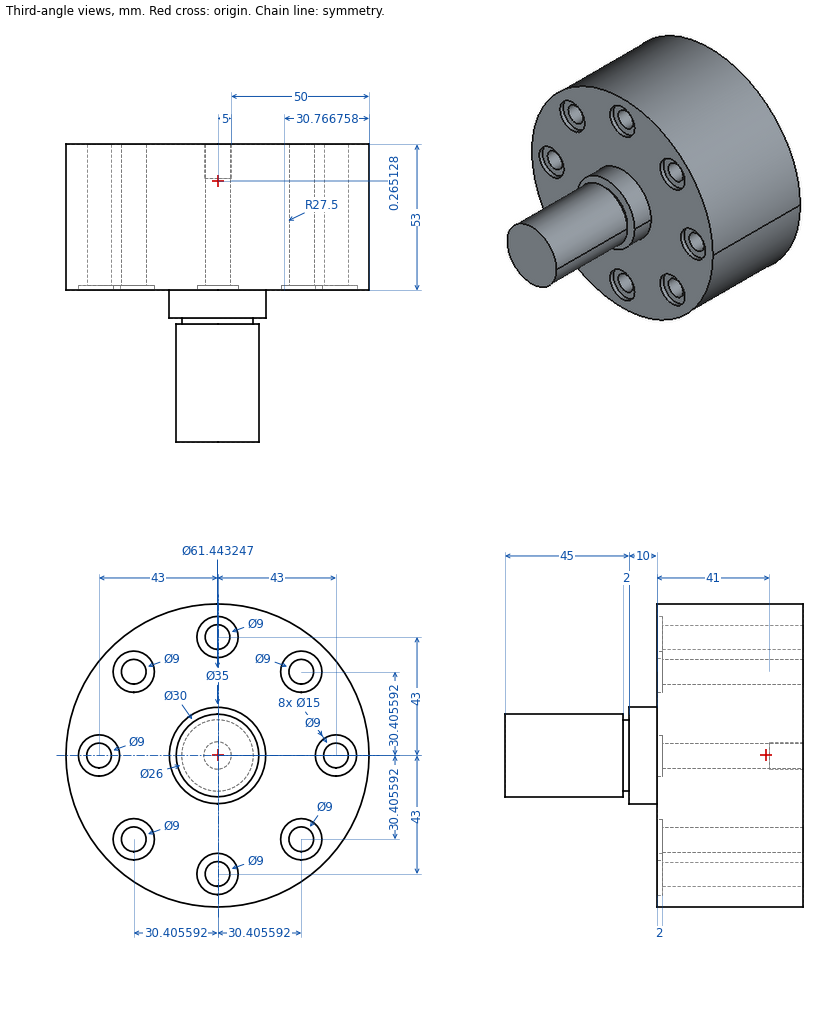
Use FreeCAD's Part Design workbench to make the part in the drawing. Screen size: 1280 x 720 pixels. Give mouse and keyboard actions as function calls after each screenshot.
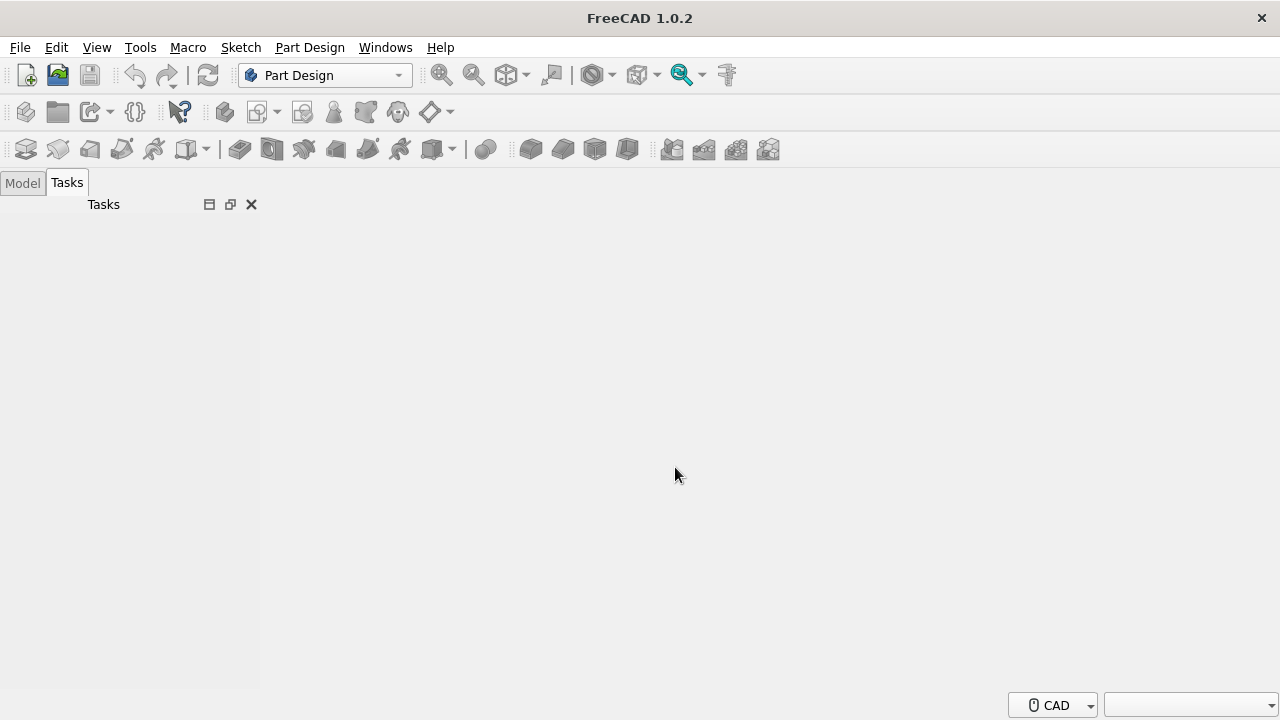
click(26, 76)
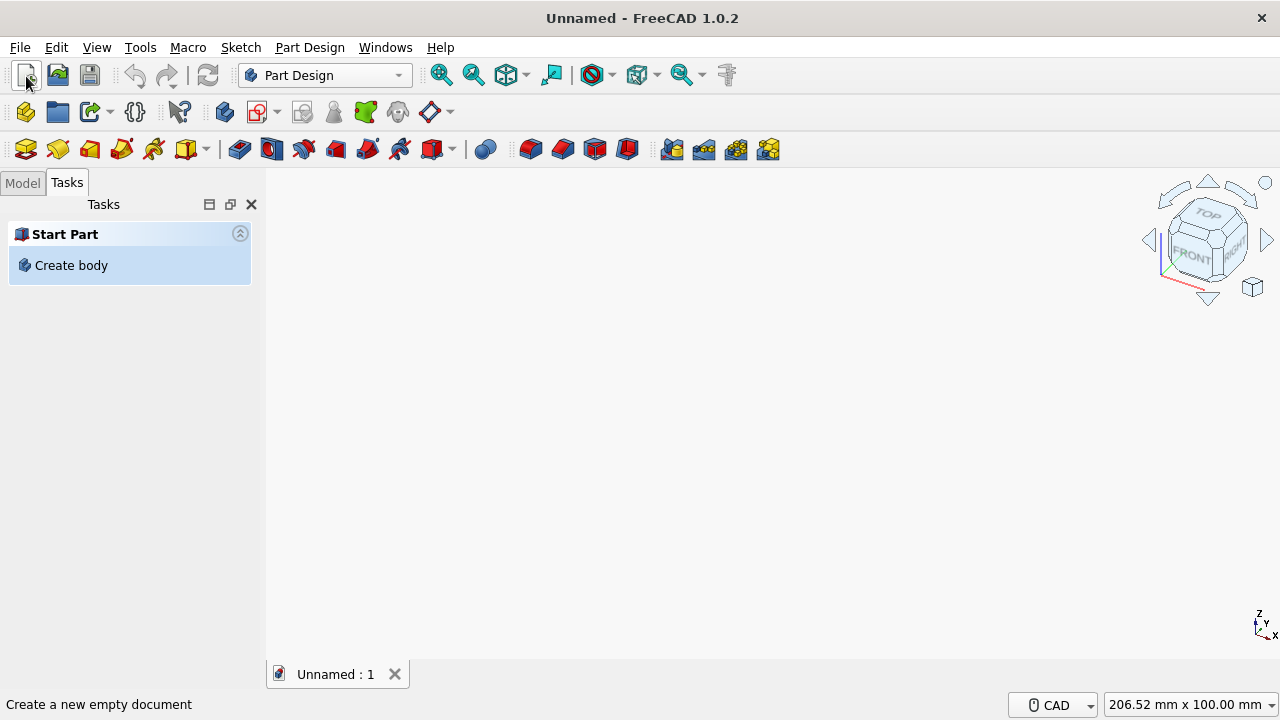
click(258, 112)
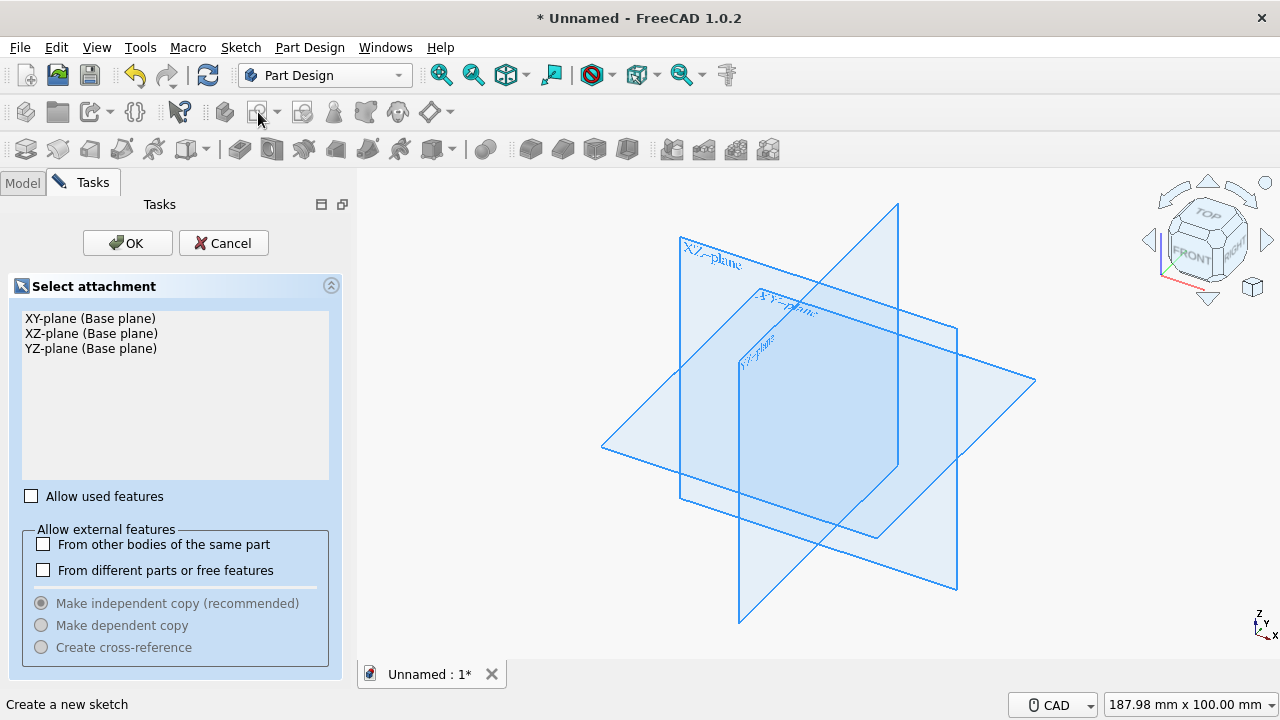
click(82, 318)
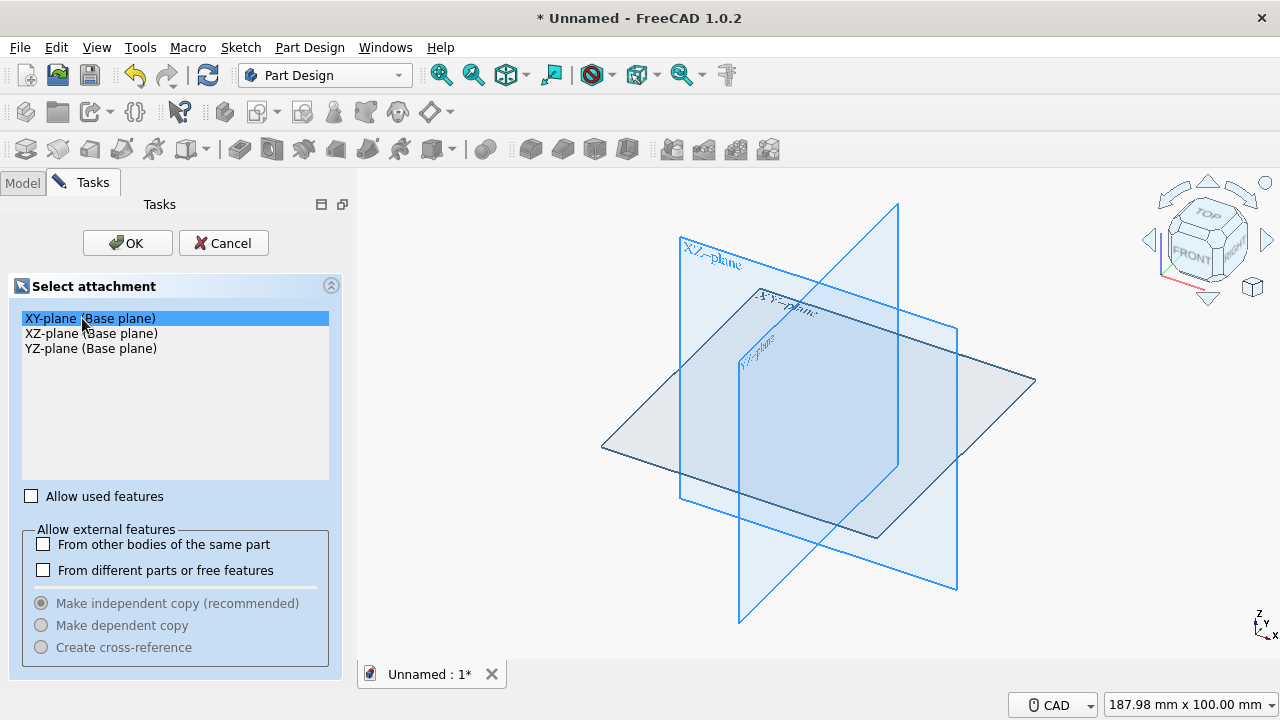
click(128, 243)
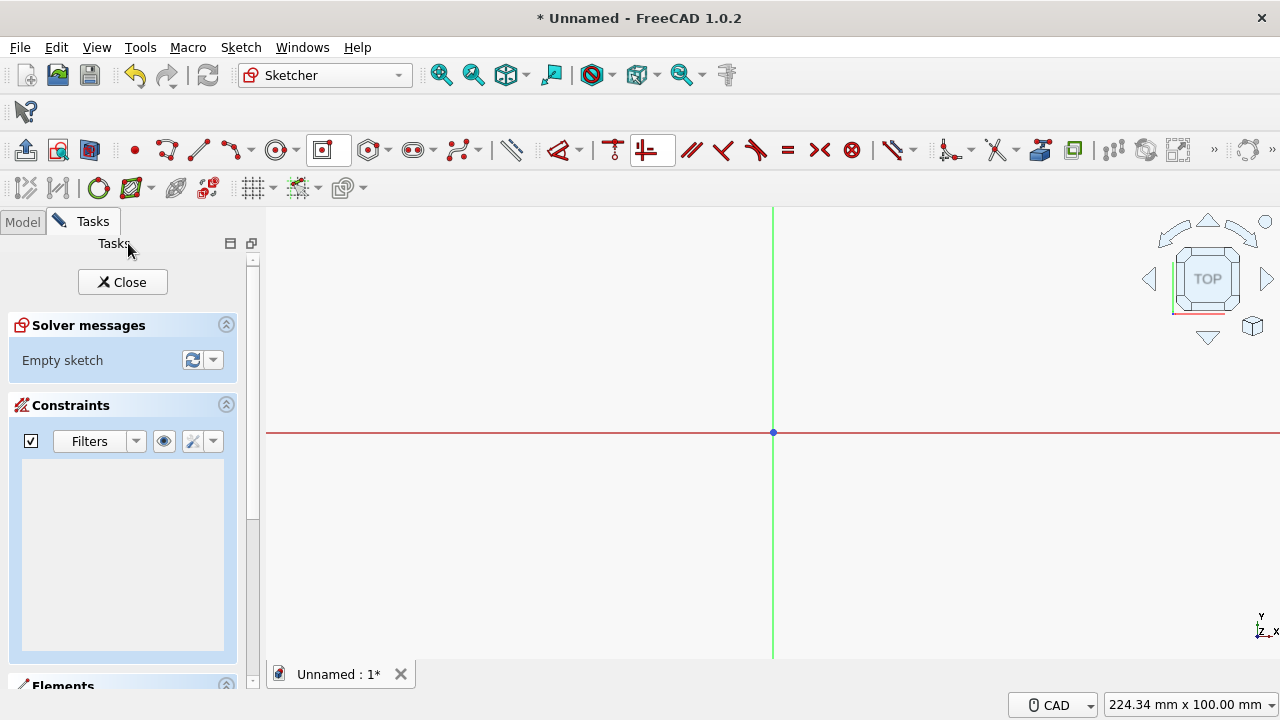
scroll(294, 235, down, 1)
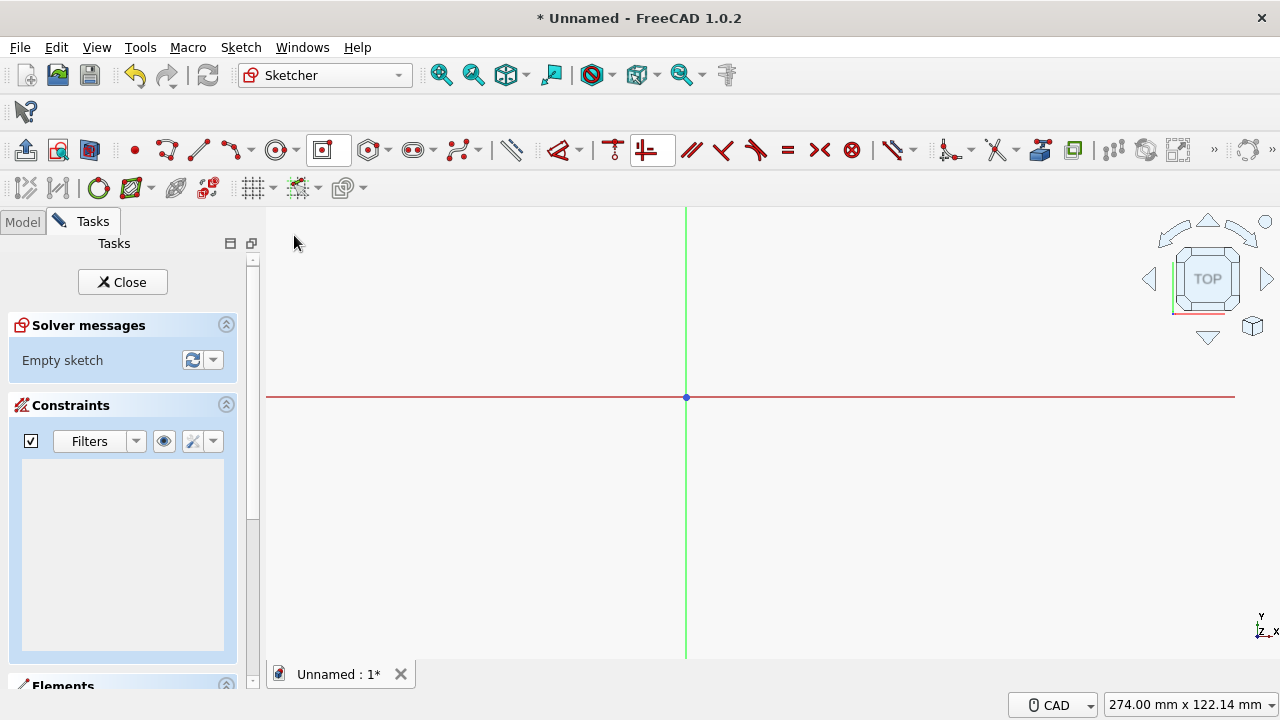
scroll(958, 473, up, 2)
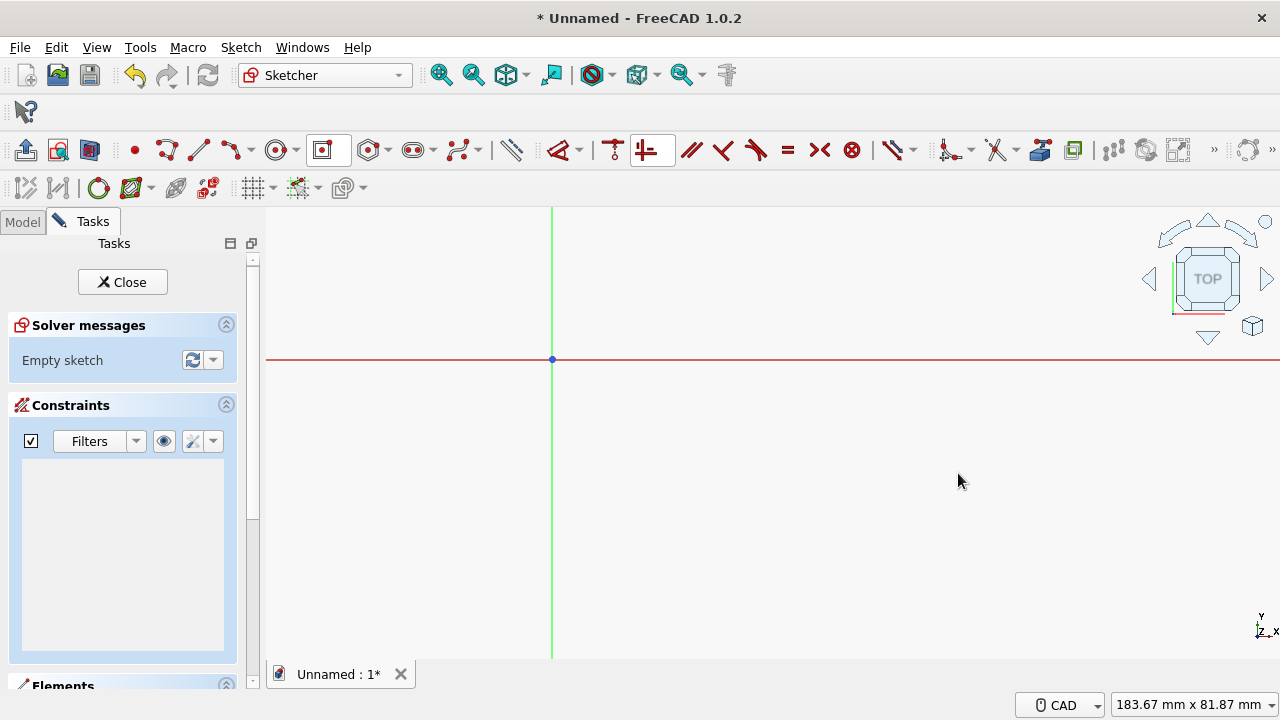
click(168, 150)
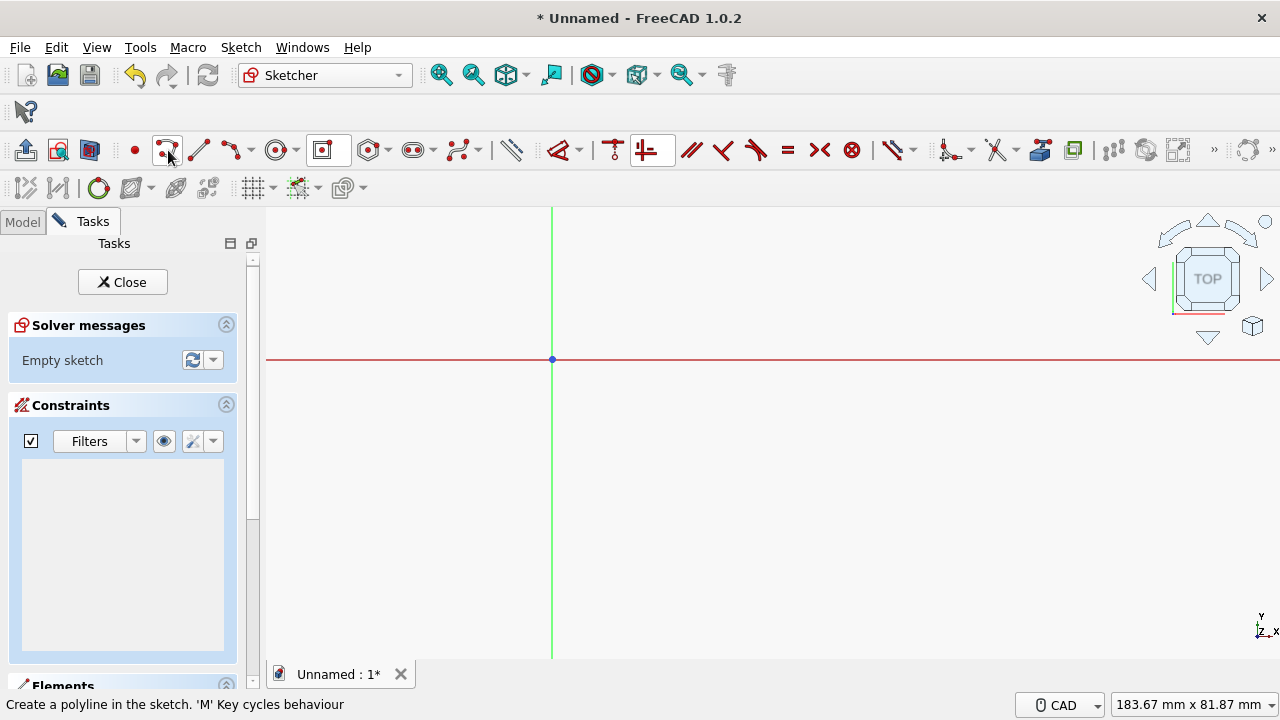
click(686, 579)
click(856, 579)
click(856, 287)
click(580, 287)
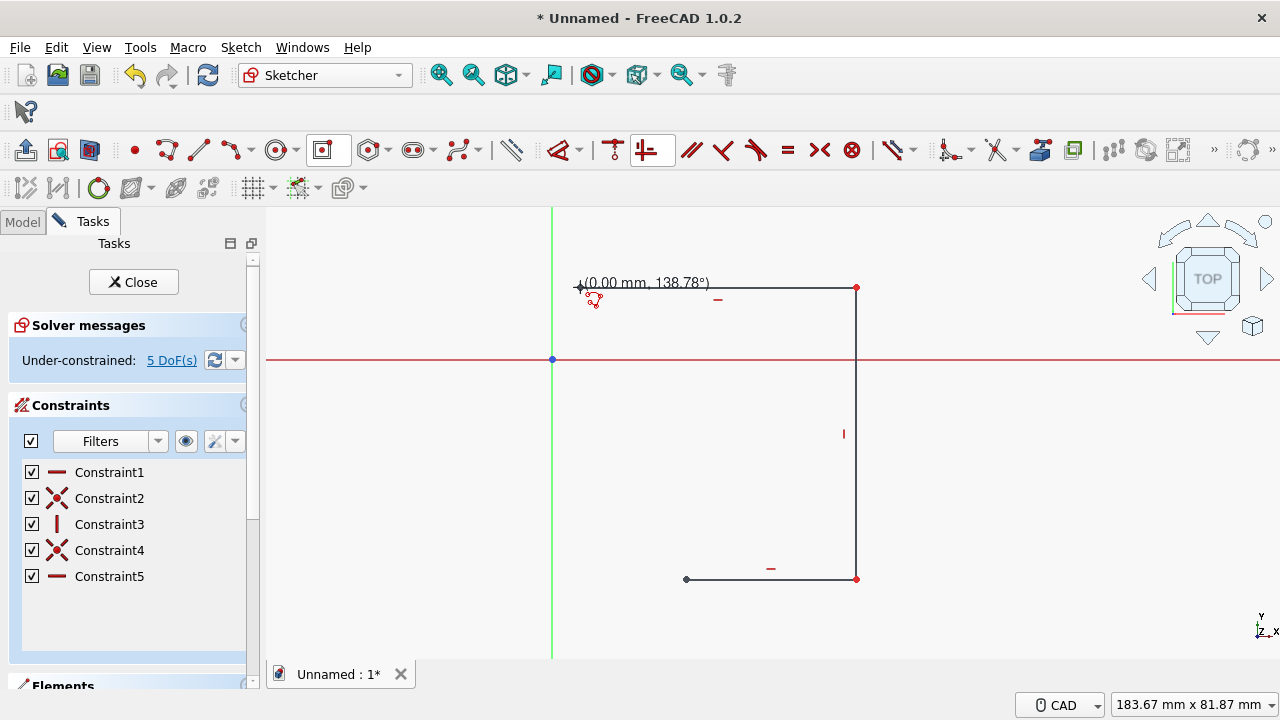
scroll(580, 358, up, 12)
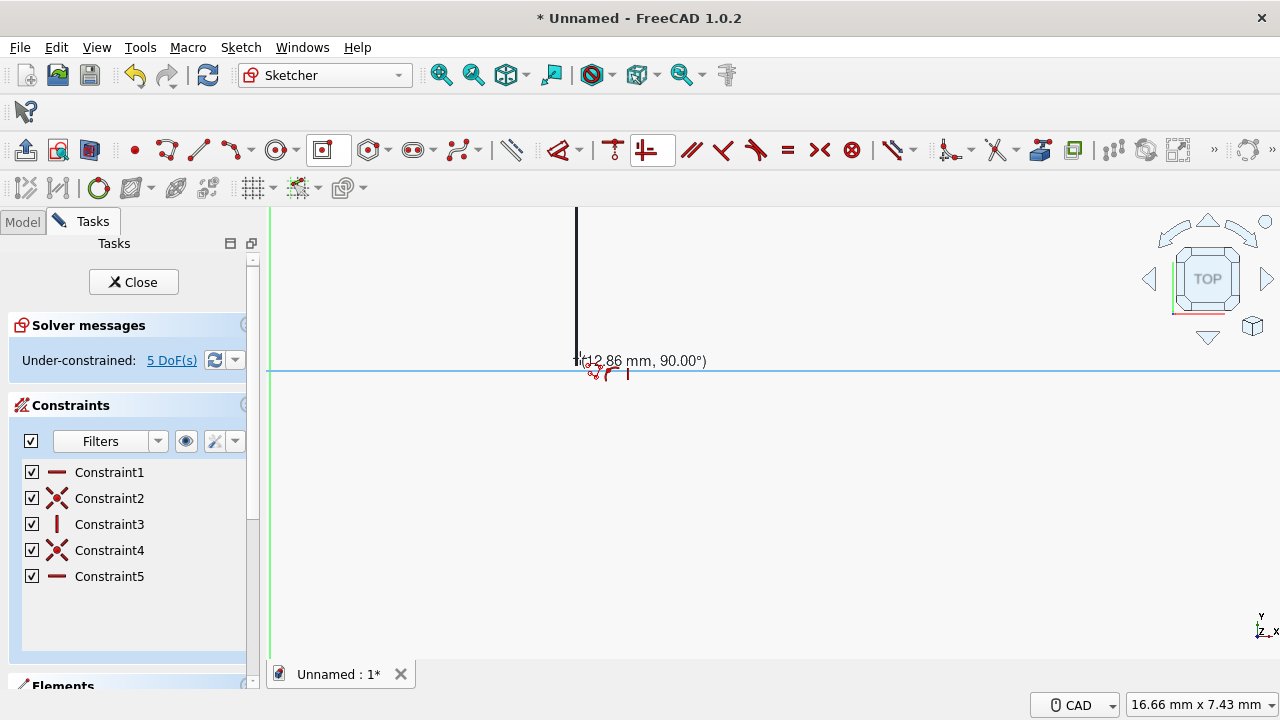
click(577, 355)
right_click(577, 355)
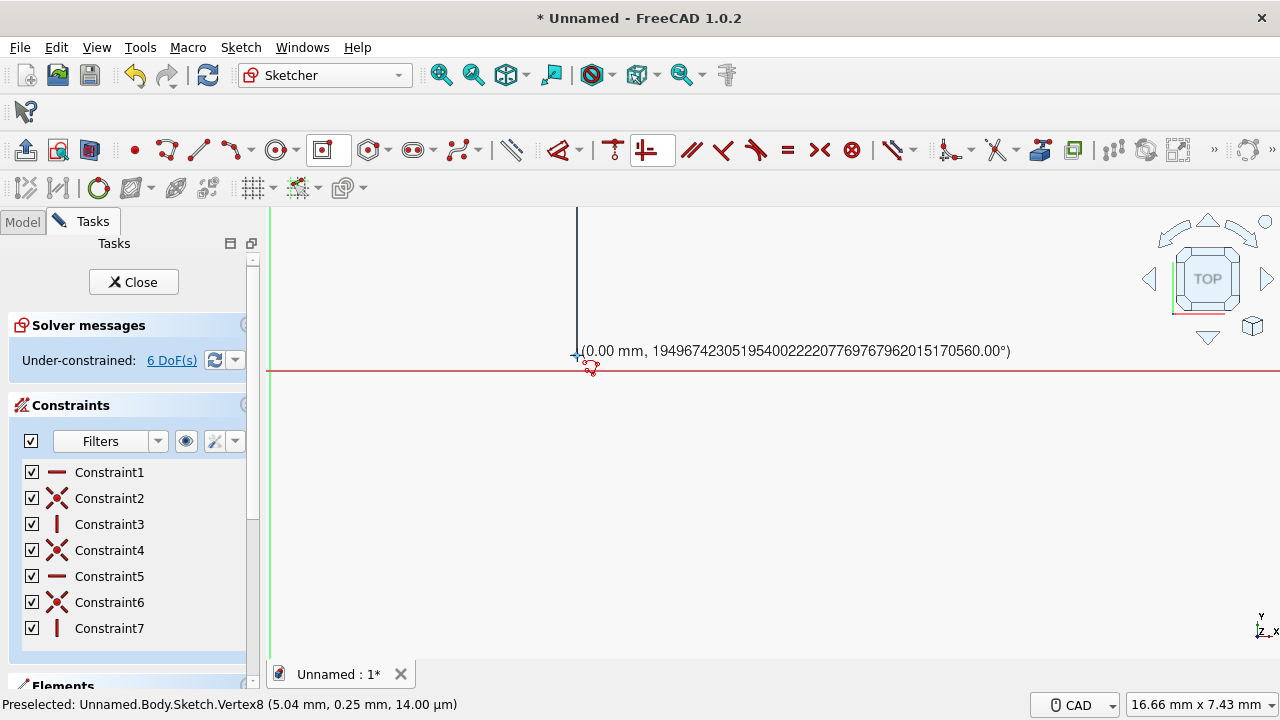
click(232, 150)